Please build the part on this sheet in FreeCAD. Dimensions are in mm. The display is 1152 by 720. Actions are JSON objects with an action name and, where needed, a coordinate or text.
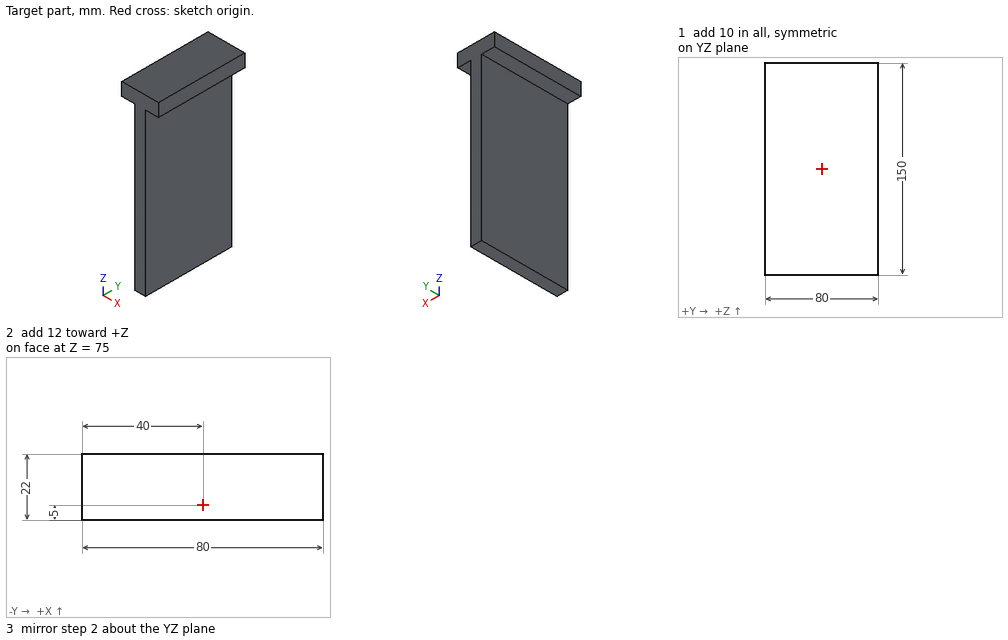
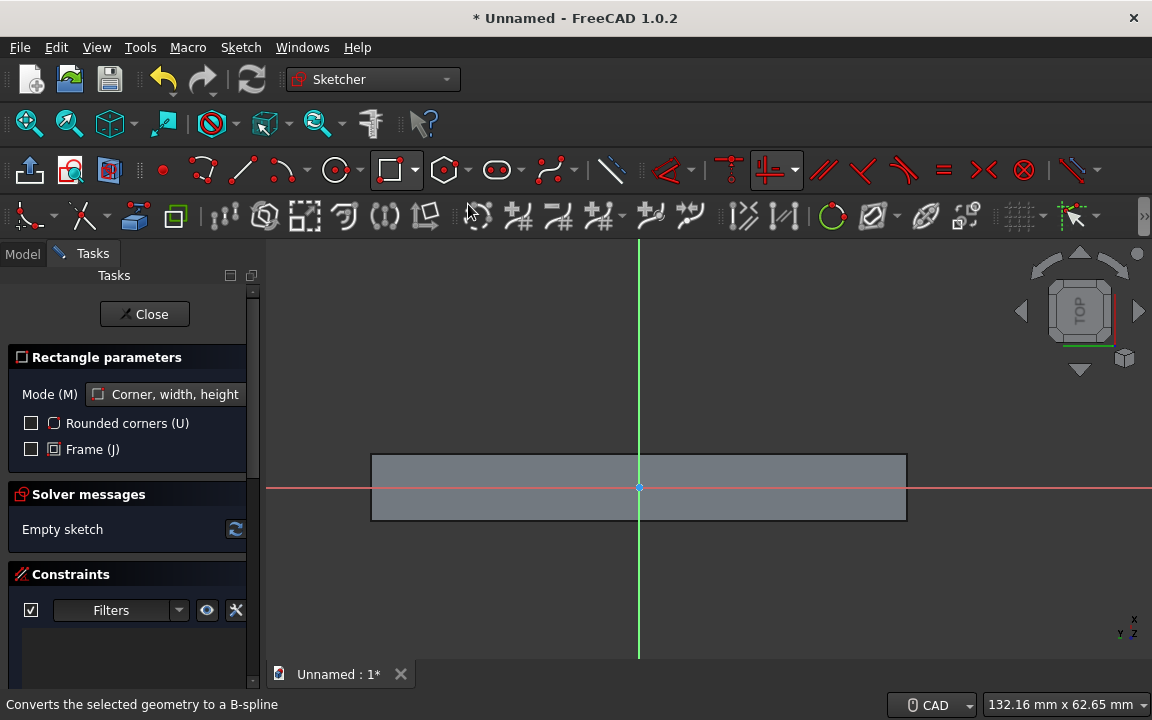
{"action": "left_click", "coordinate": [371, 374]}
{"action": "left_click", "coordinate": [907, 521]}
{"action": "key", "text": "Escape"}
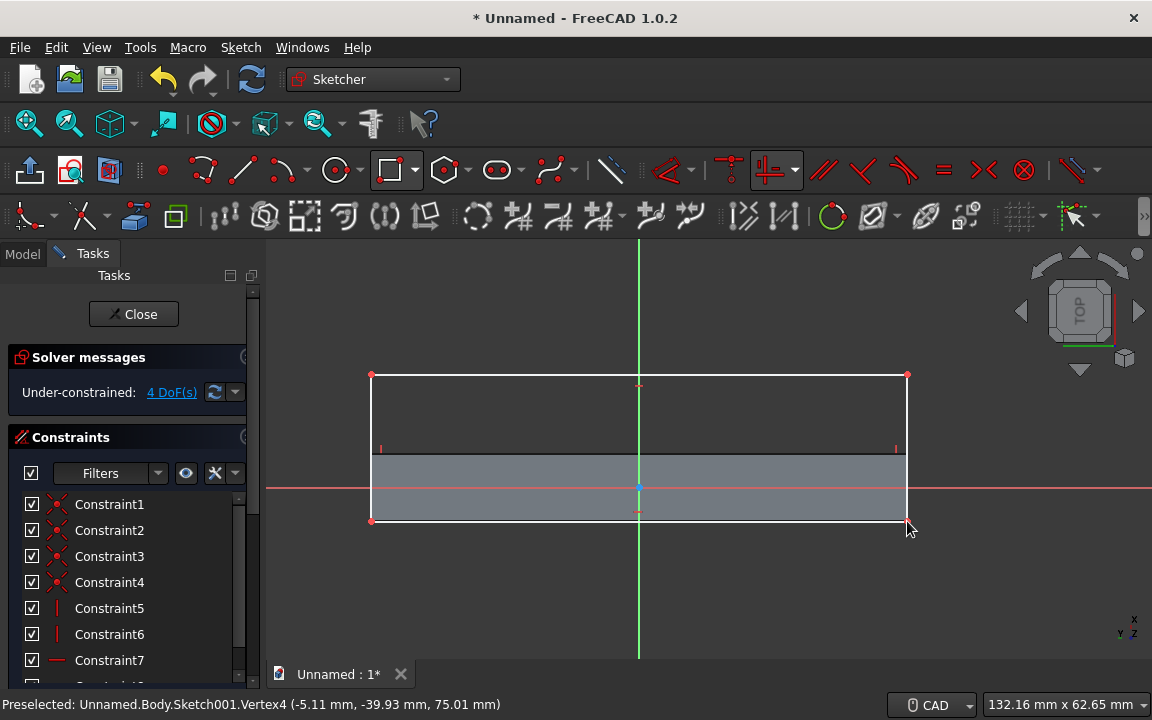
{"action": "left_click", "coordinate": [666, 170]}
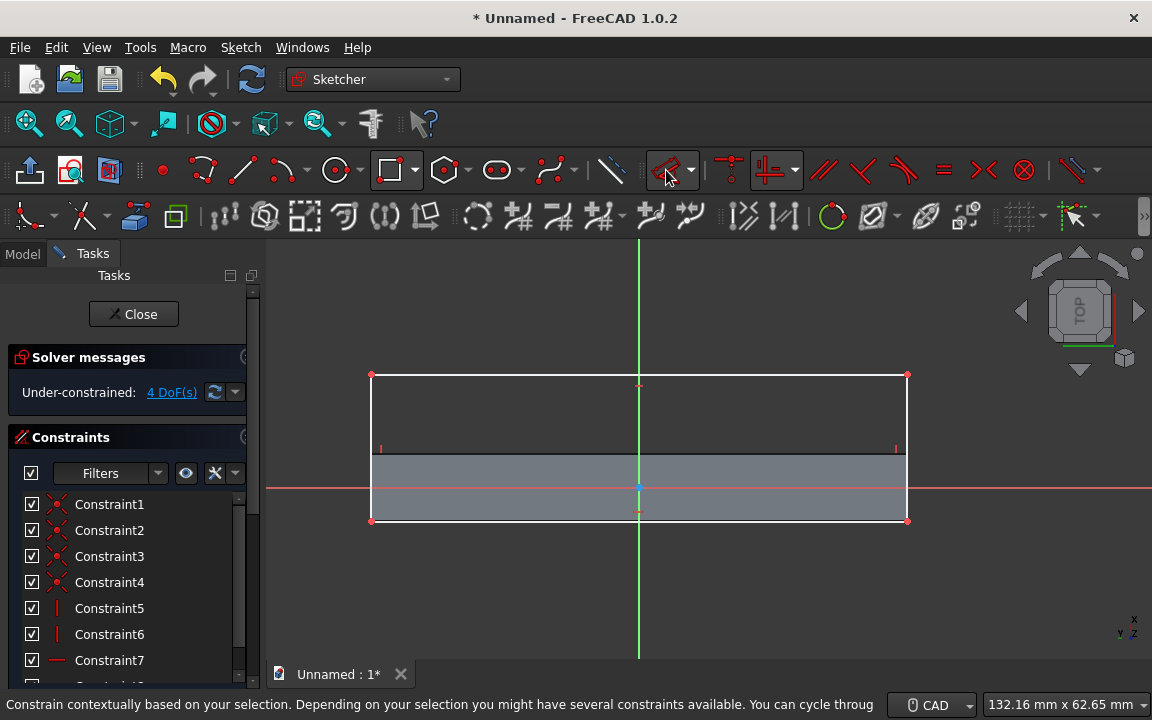
{"action": "left_click", "coordinate": [371, 419]}
{"action": "left_click", "coordinate": [337, 448]}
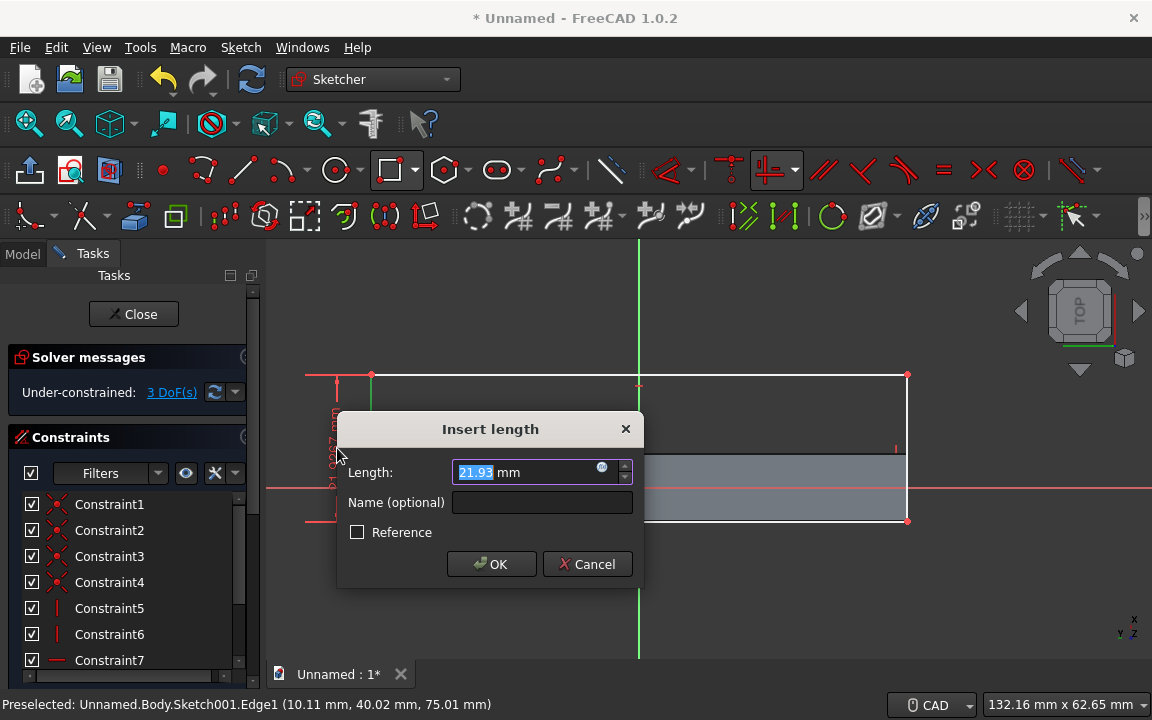
{"action": "type", "text": "22"}
{"action": "key", "text": "Return"}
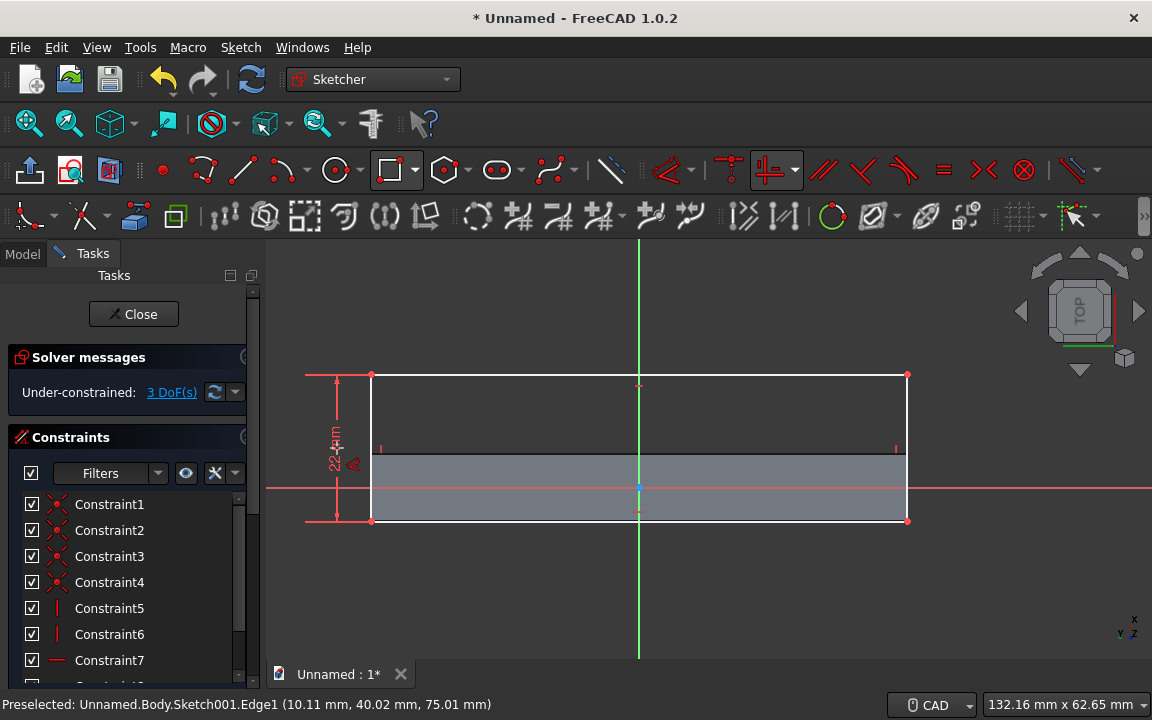
{"action": "left_click", "coordinate": [532, 522]}
{"action": "left_click", "coordinate": [516, 556]}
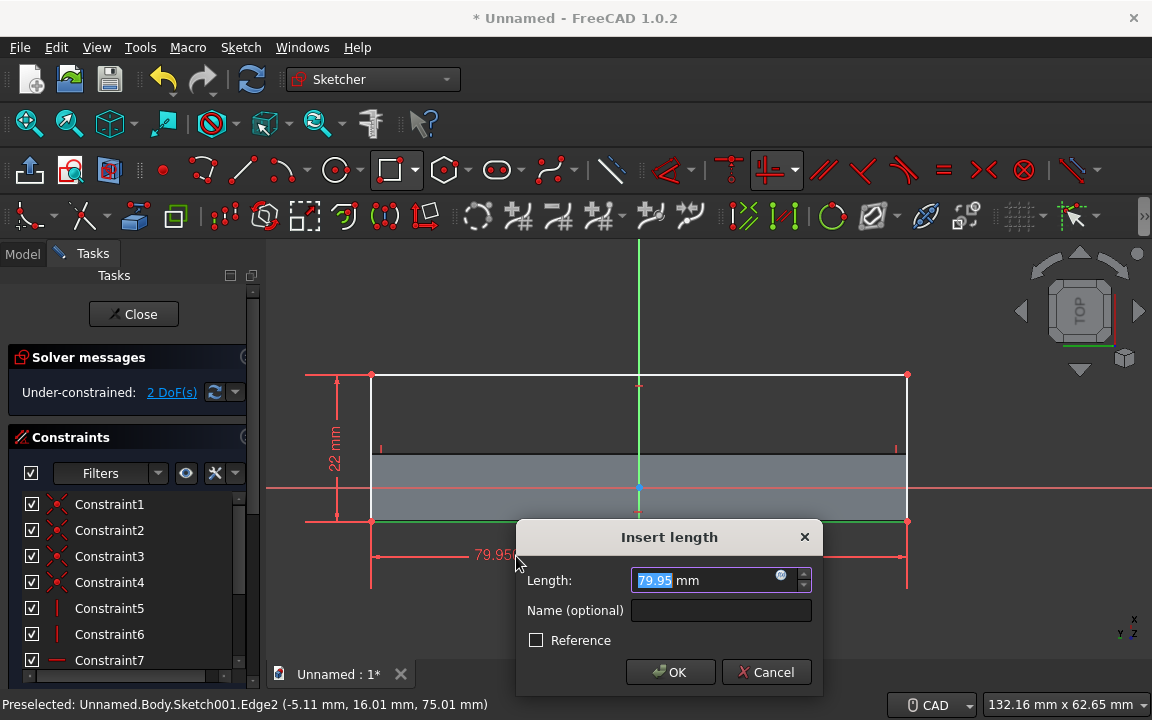
{"action": "type", "text": "80"}
{"action": "key", "text": "Return"}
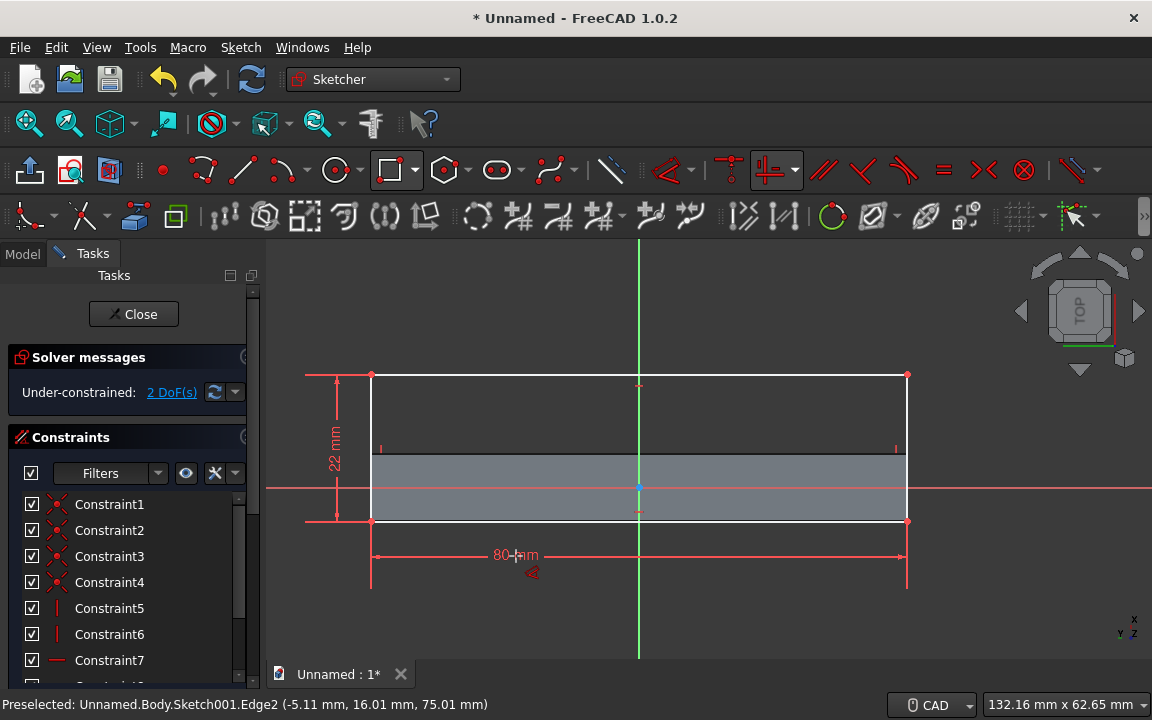
{"action": "left_click", "coordinate": [371, 522]}
{"action": "left_click", "coordinate": [337, 505]}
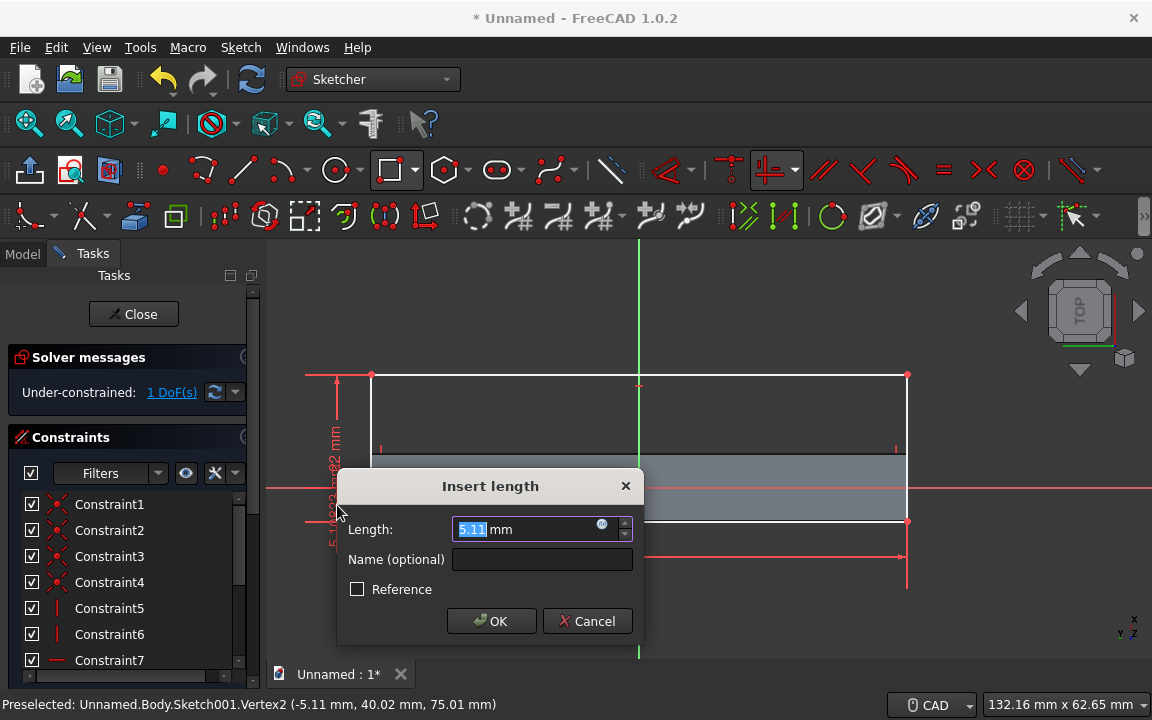
{"action": "type", "text": "5"}
{"action": "key", "text": "Return"}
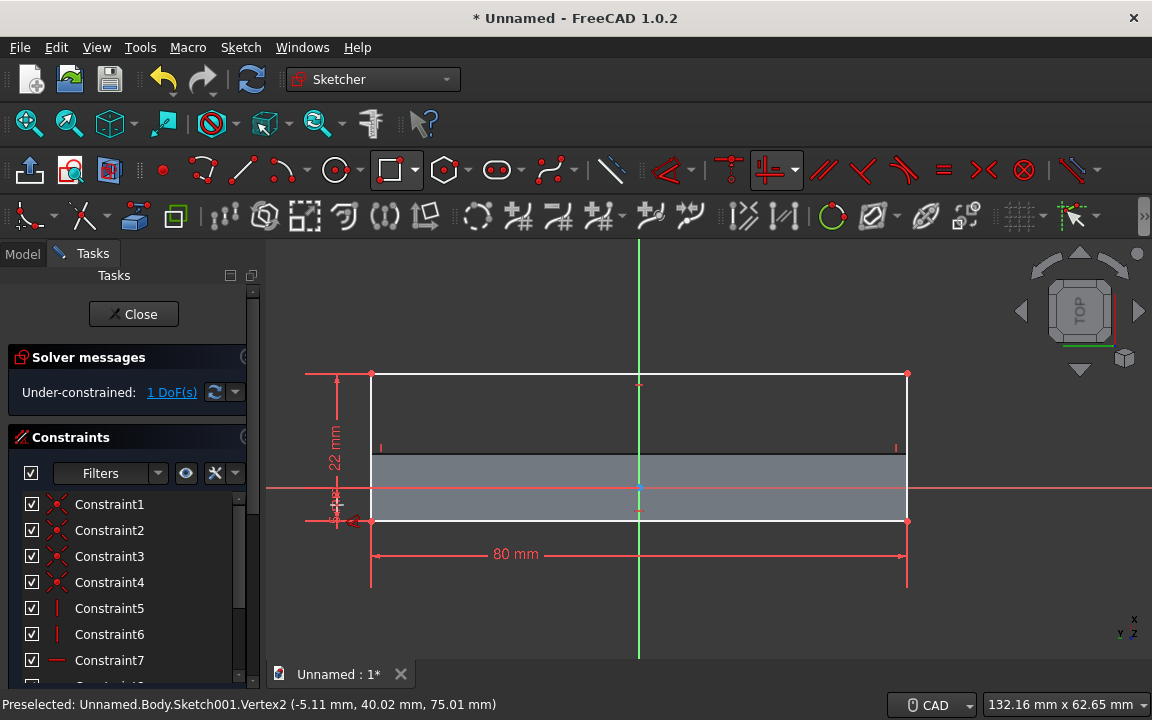
{"action": "left_click", "coordinate": [371, 374]}
{"action": "left_click", "coordinate": [505, 340]}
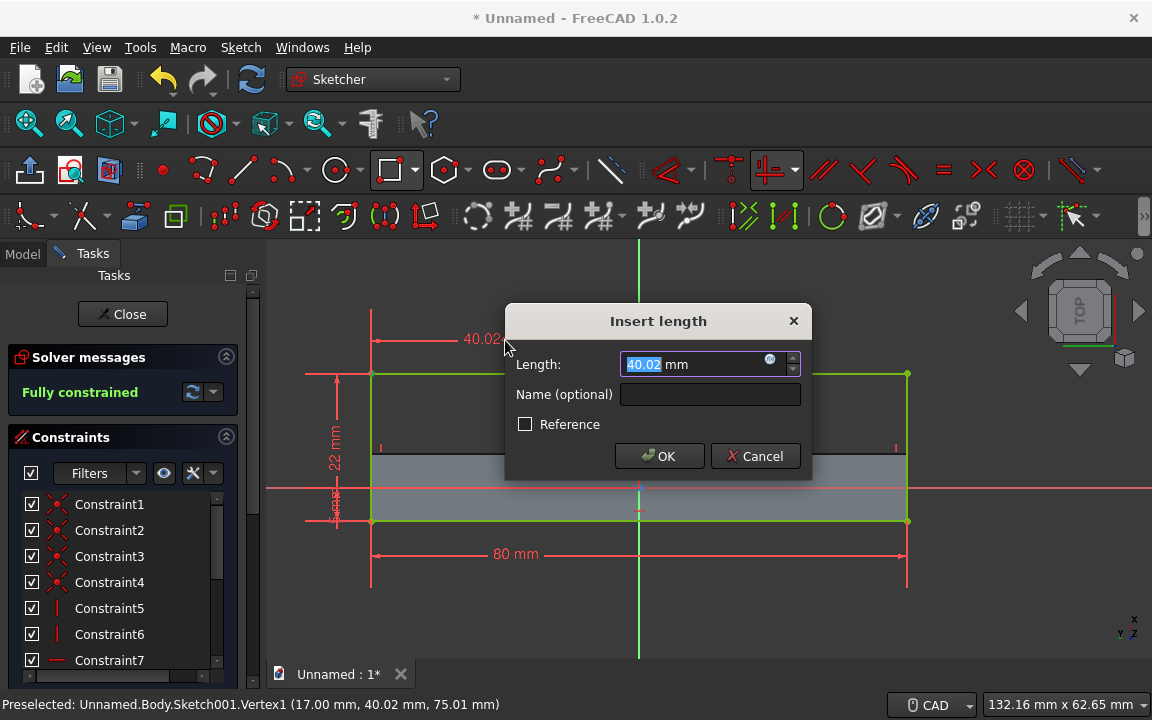
{"action": "type", "text": "40"}
{"action": "key", "text": "Return"}
{"action": "key", "text": "Escape"}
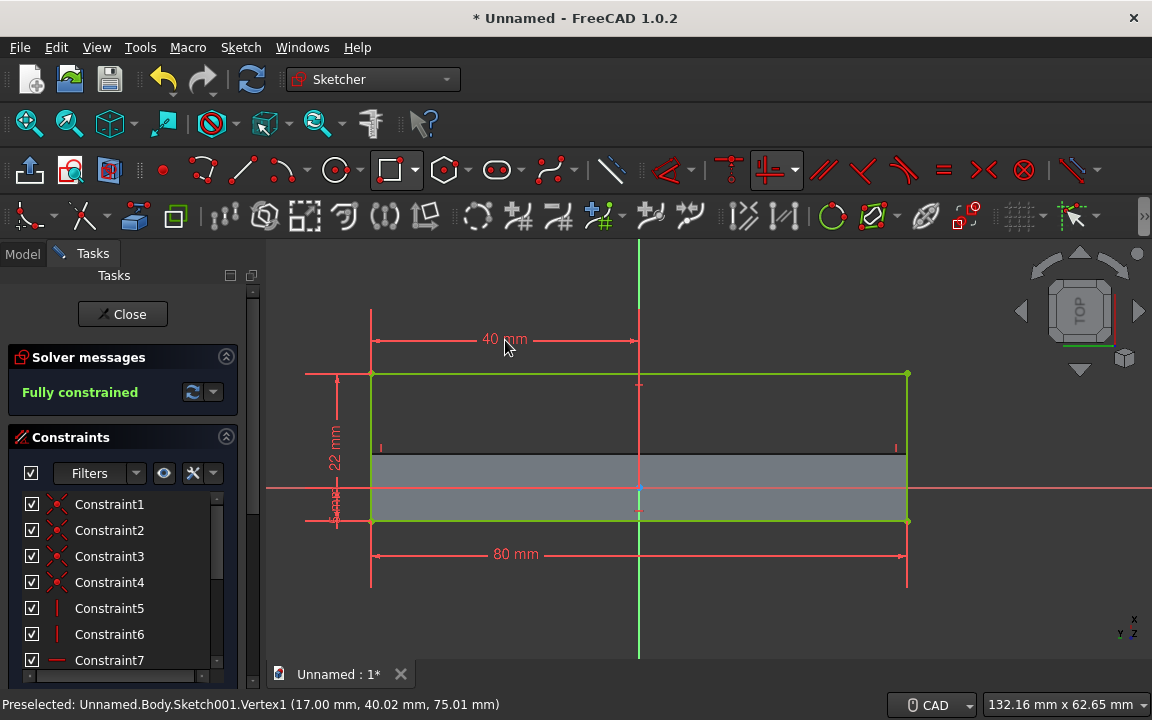
{"action": "left_click", "coordinate": [123, 314]}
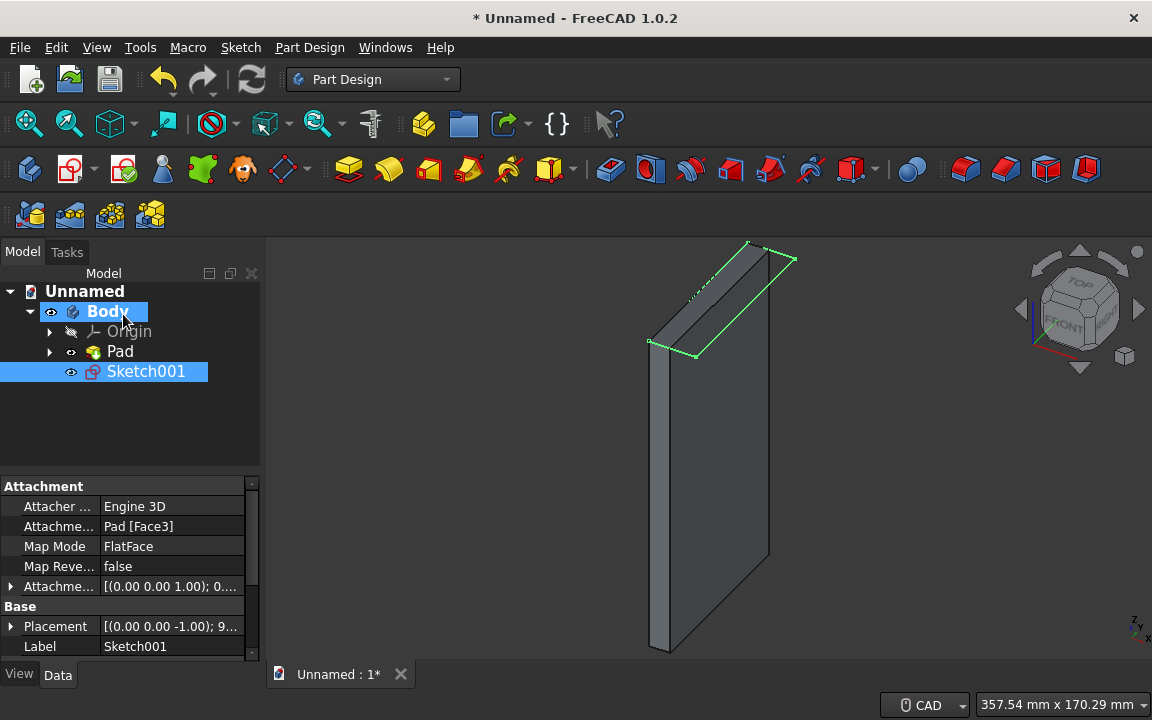
{"action": "left_click", "coordinate": [350, 170]}